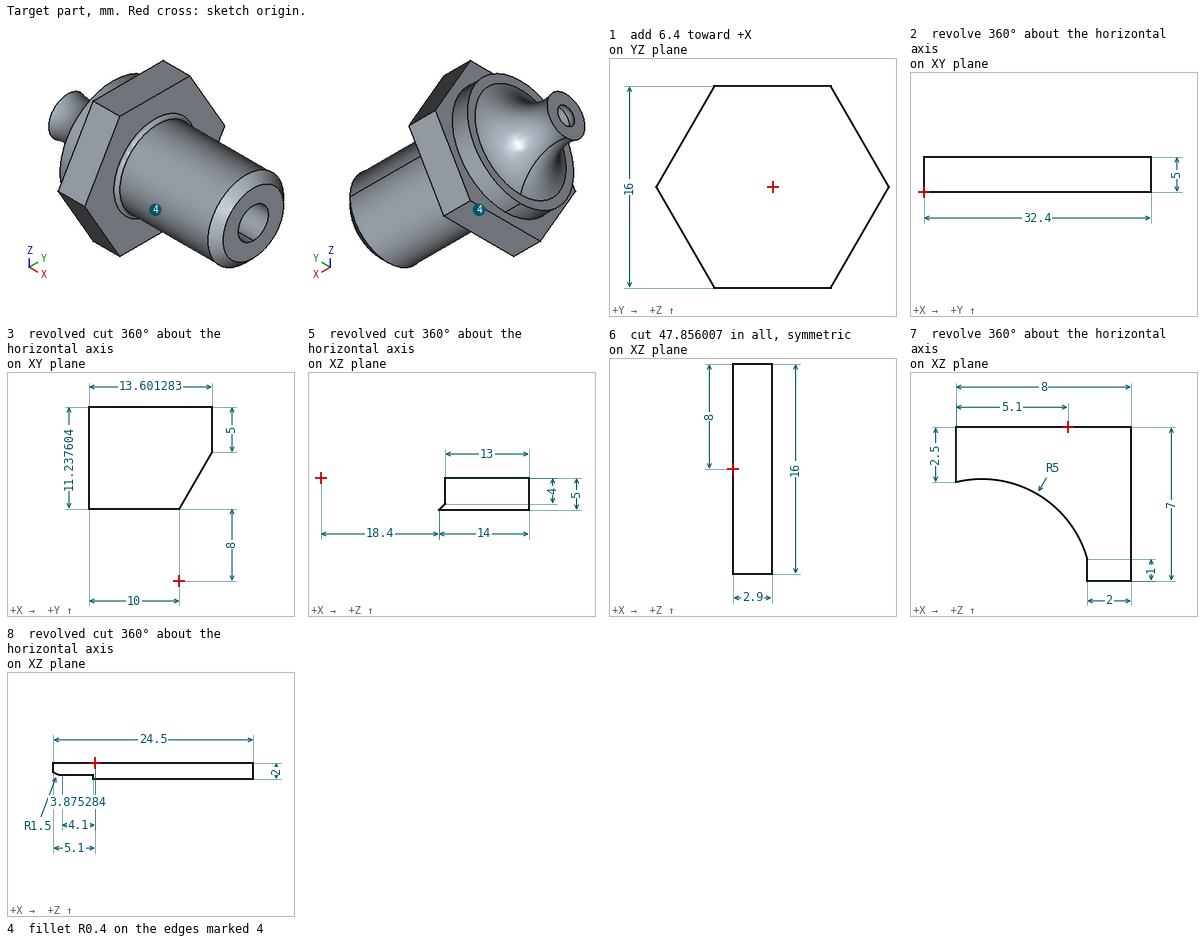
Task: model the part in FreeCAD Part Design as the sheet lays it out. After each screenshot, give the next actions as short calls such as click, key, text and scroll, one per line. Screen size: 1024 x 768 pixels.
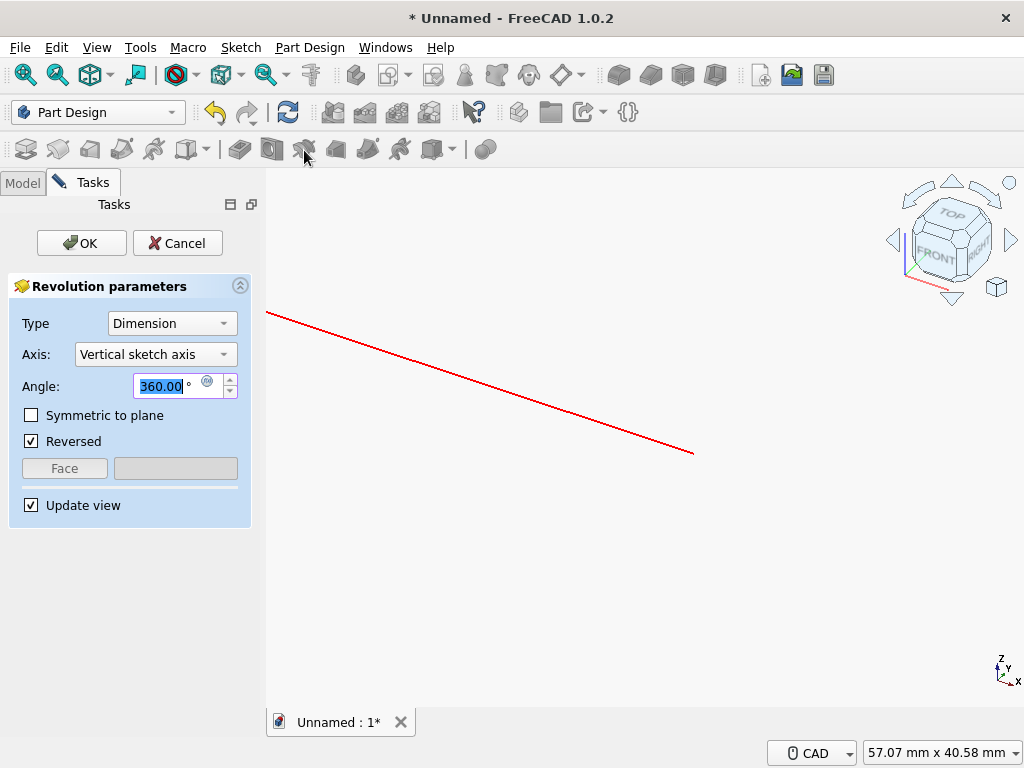
click(156, 354)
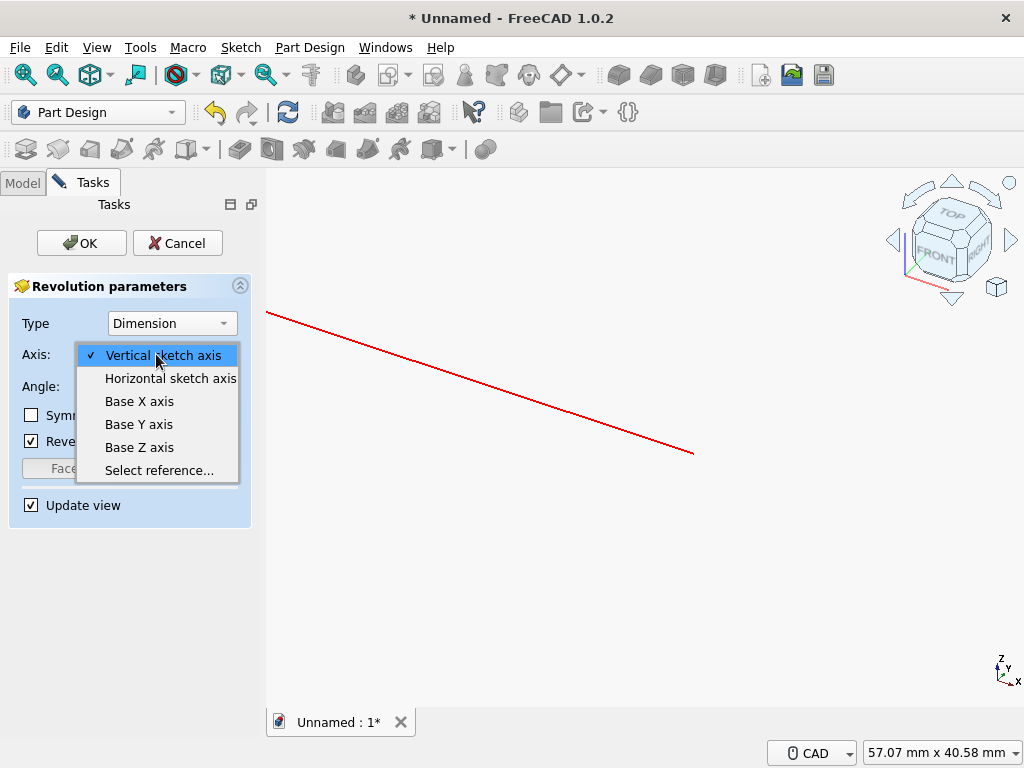
click(156, 378)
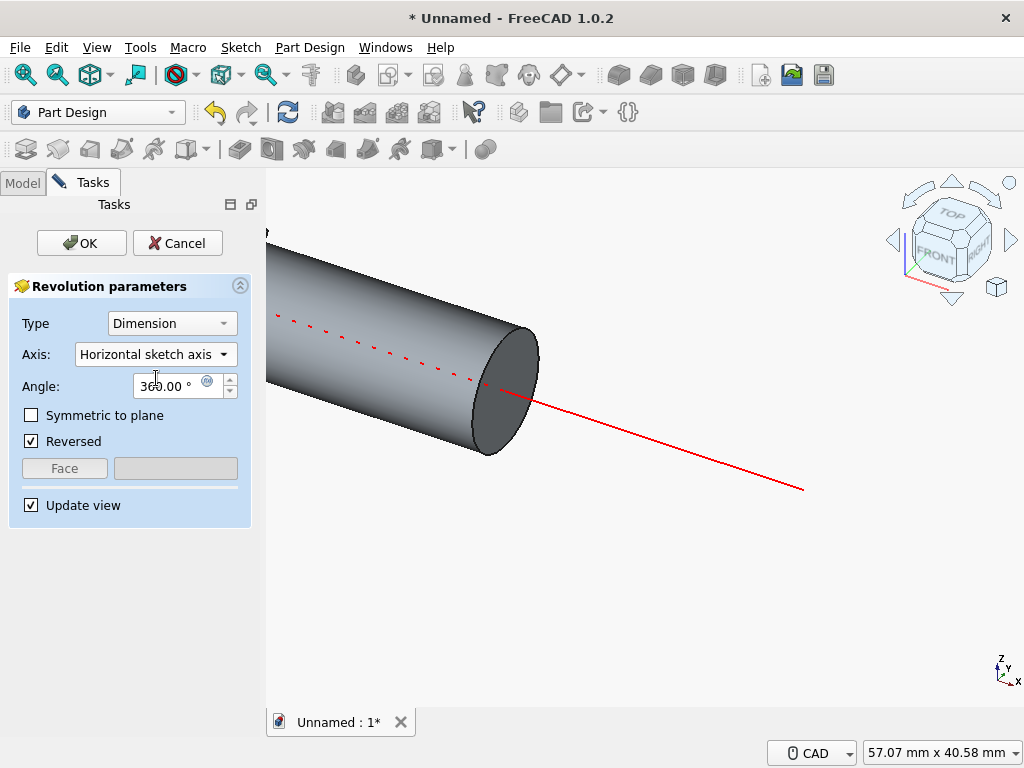
click(82, 243)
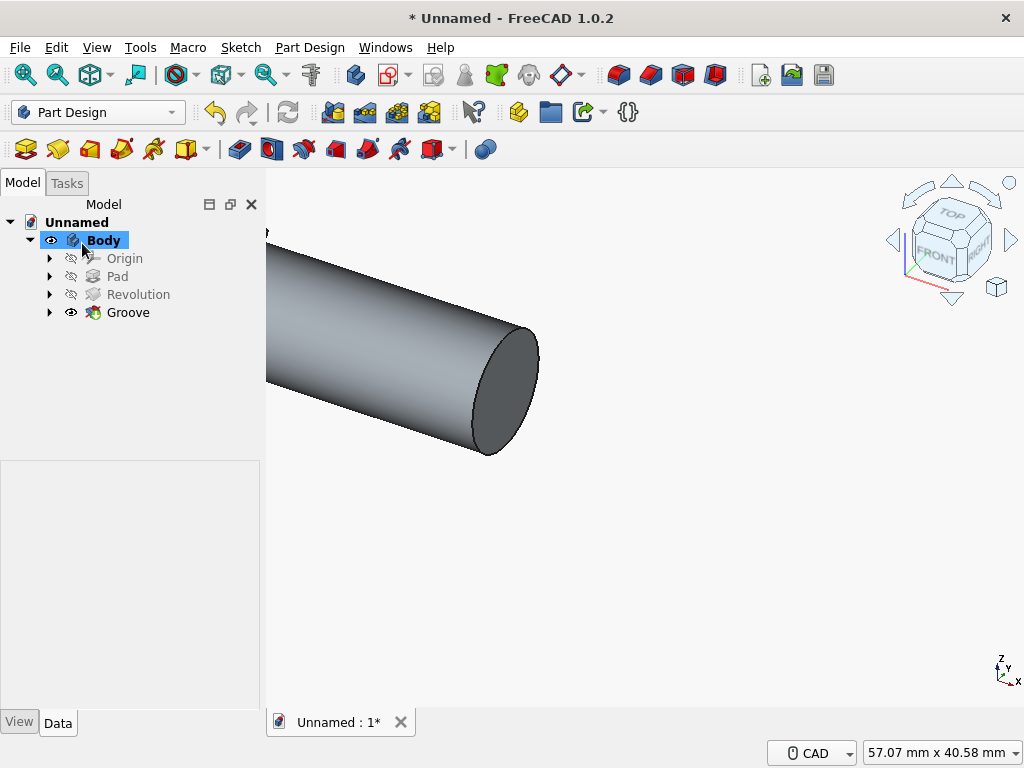
click(26, 76)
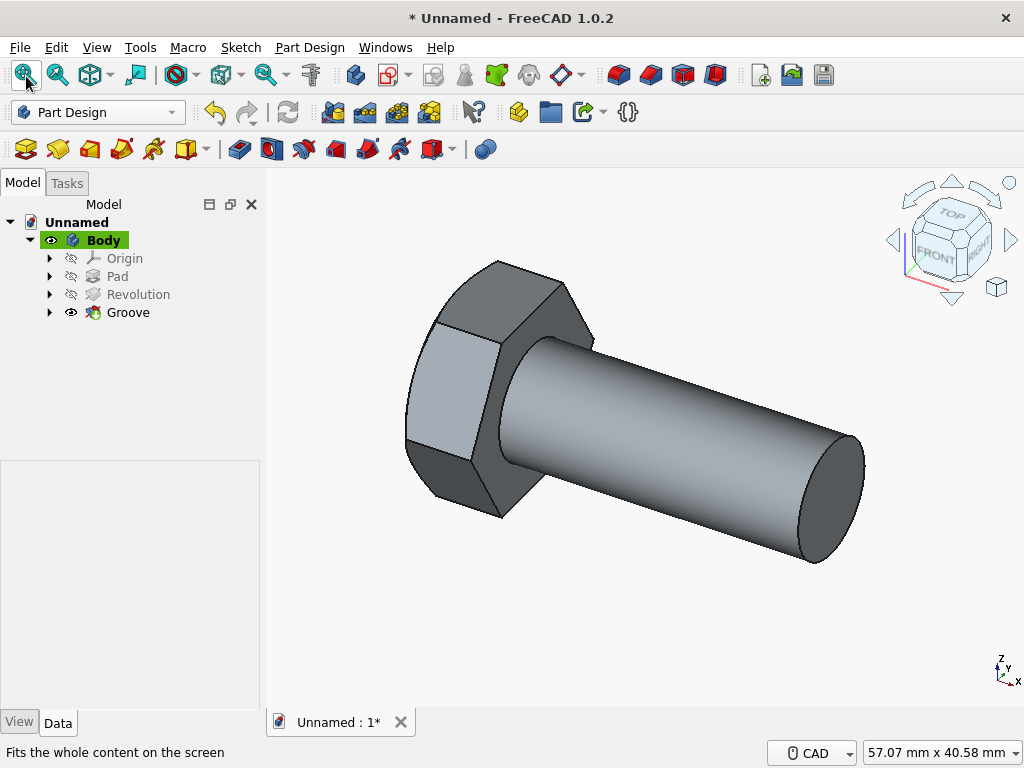
key(0)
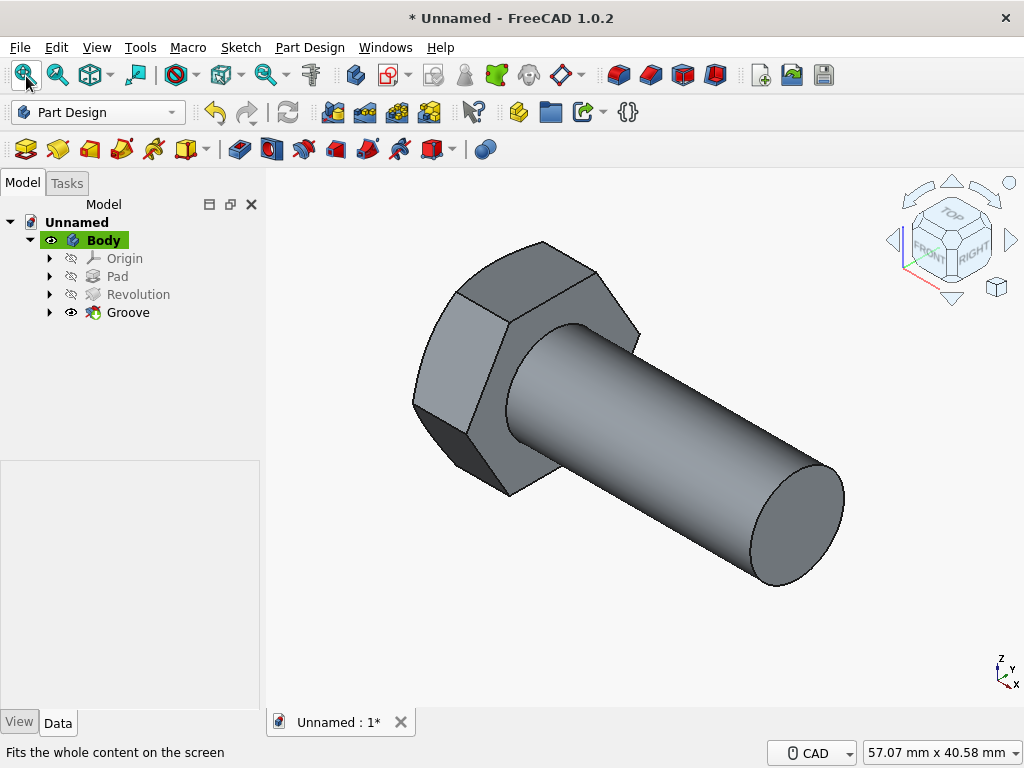
key(2)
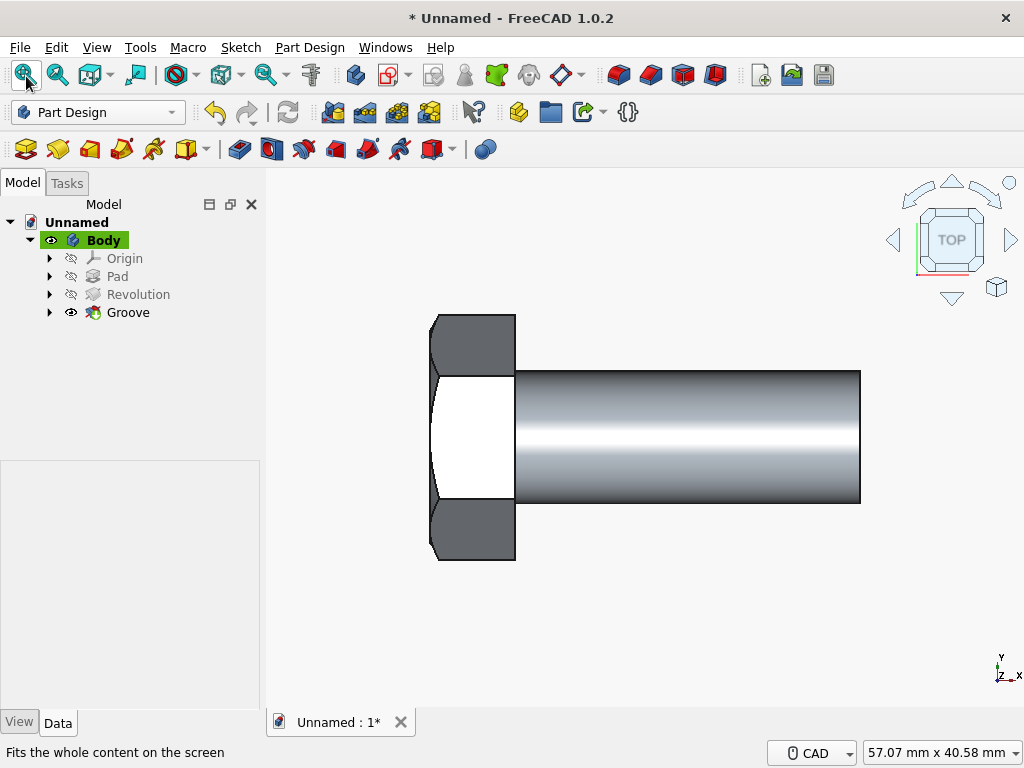
key(1)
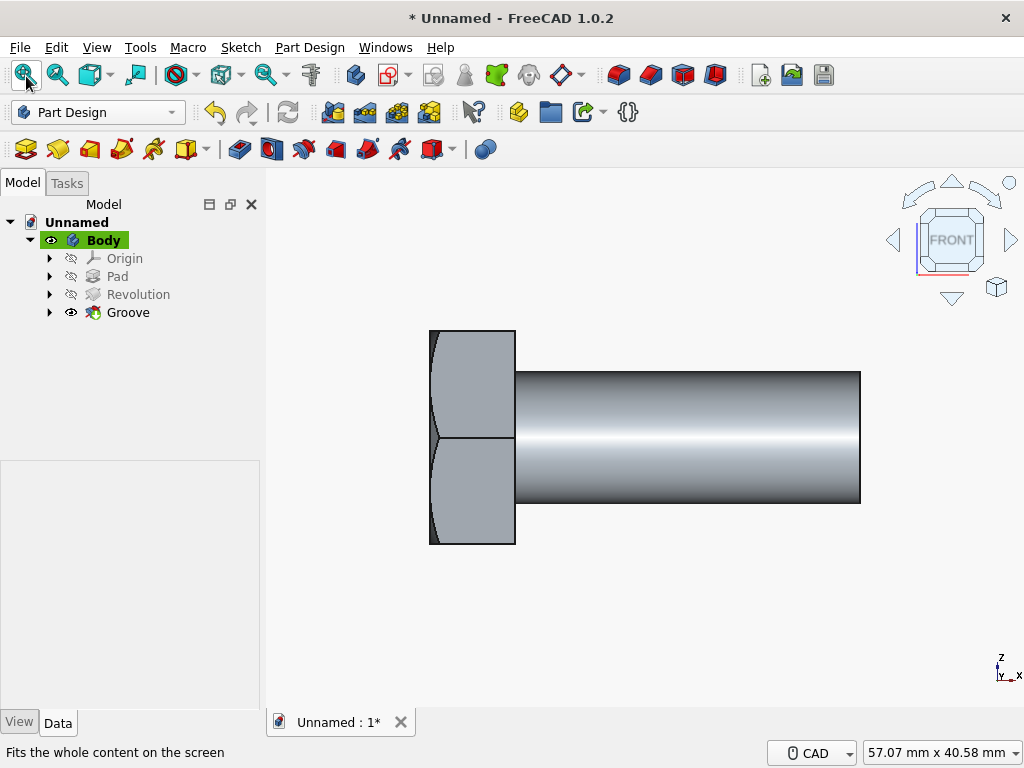
key(3)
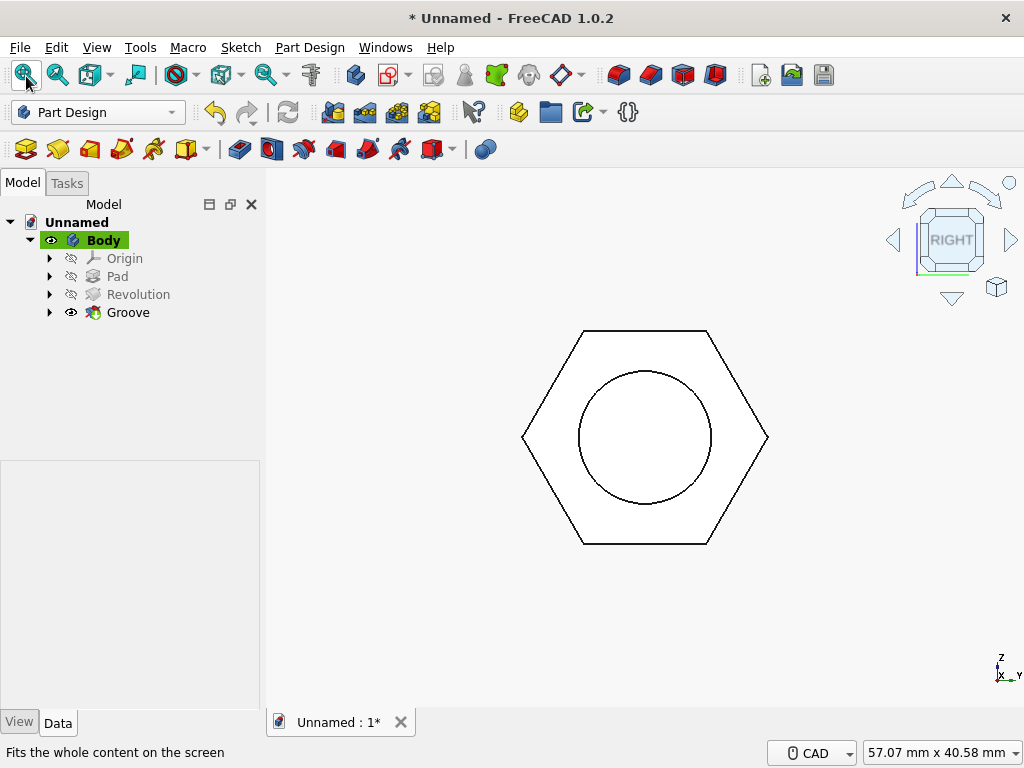
click(26, 76)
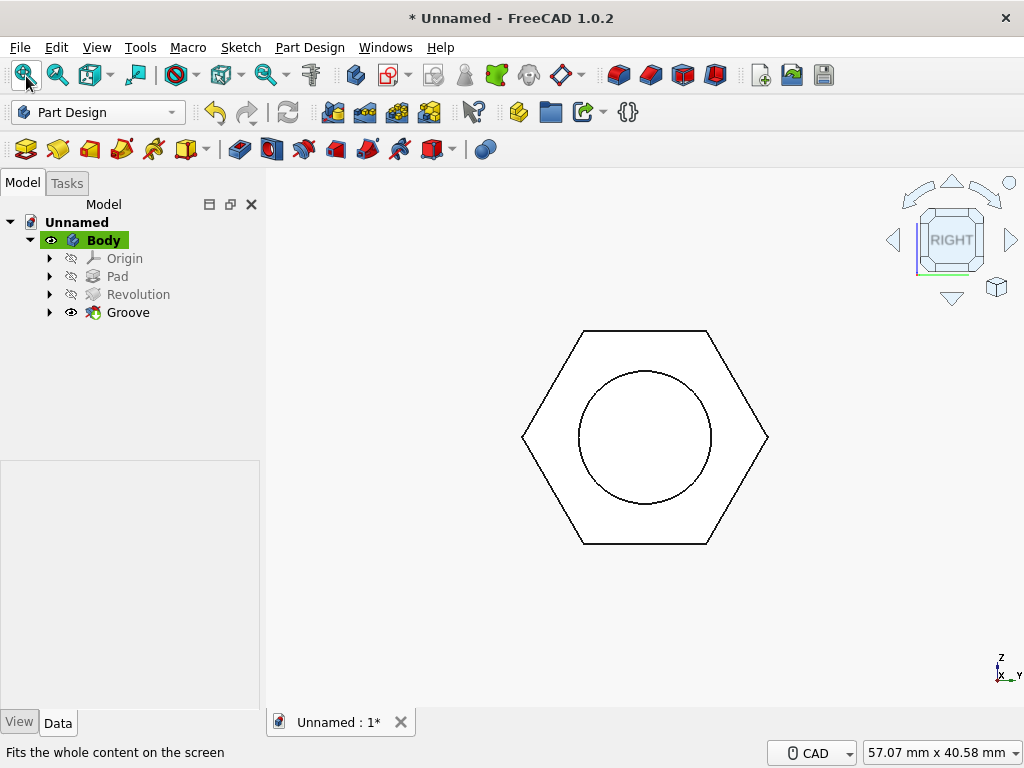
key(5)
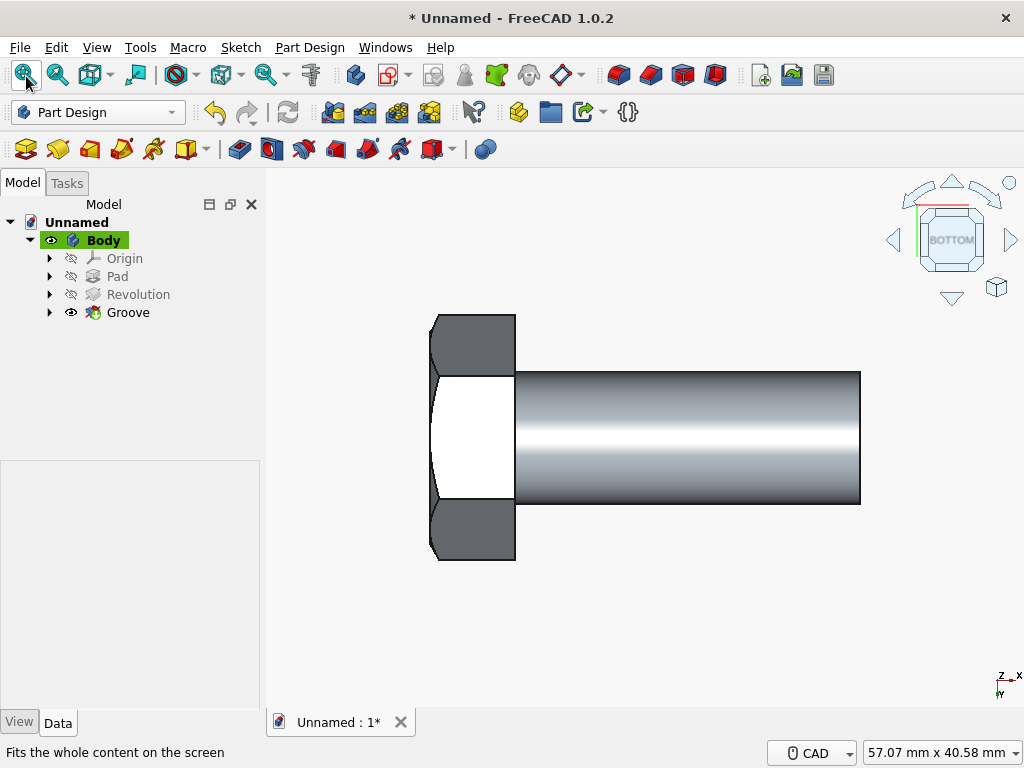
key(4)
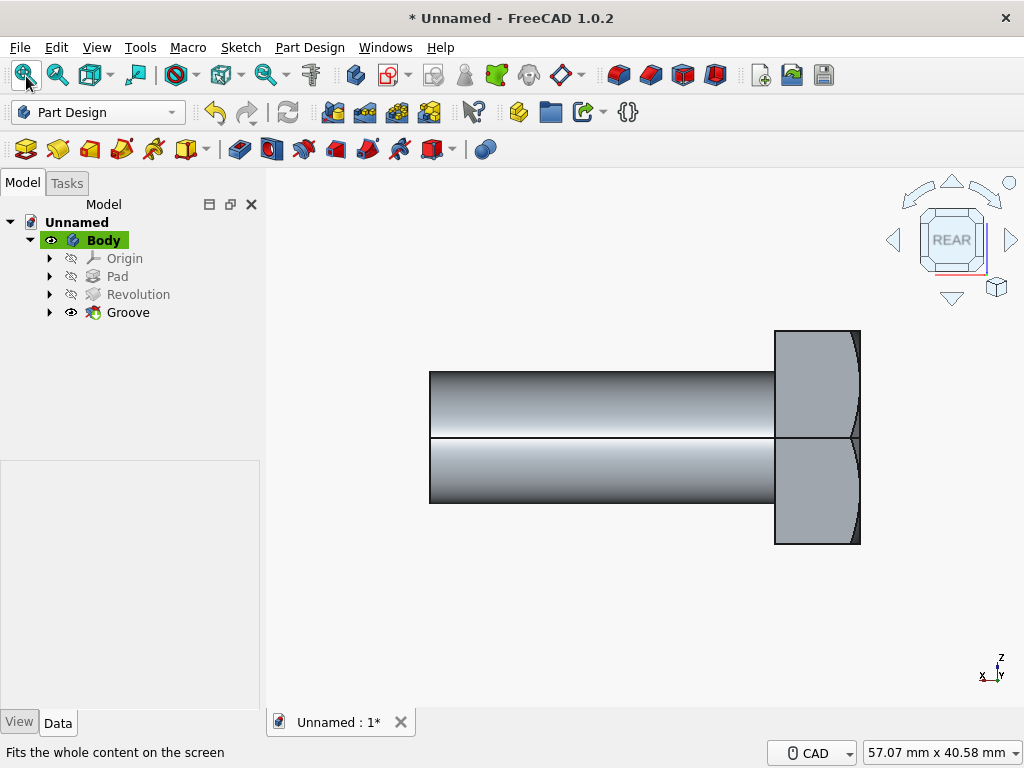
key(6)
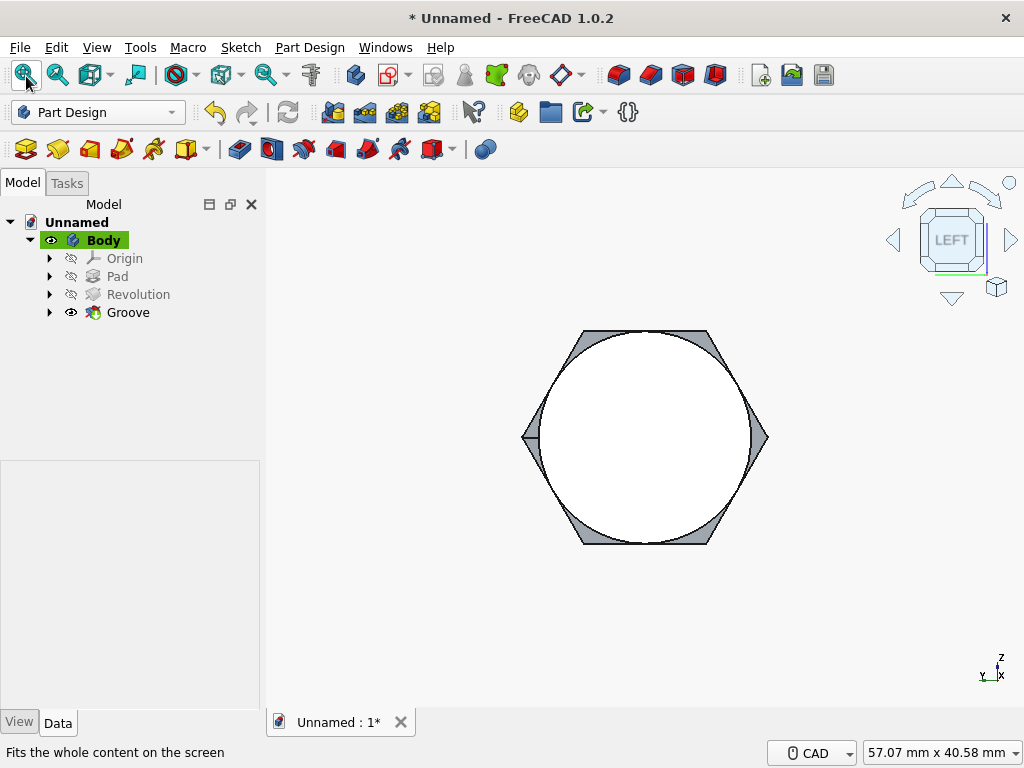
click(26, 76)